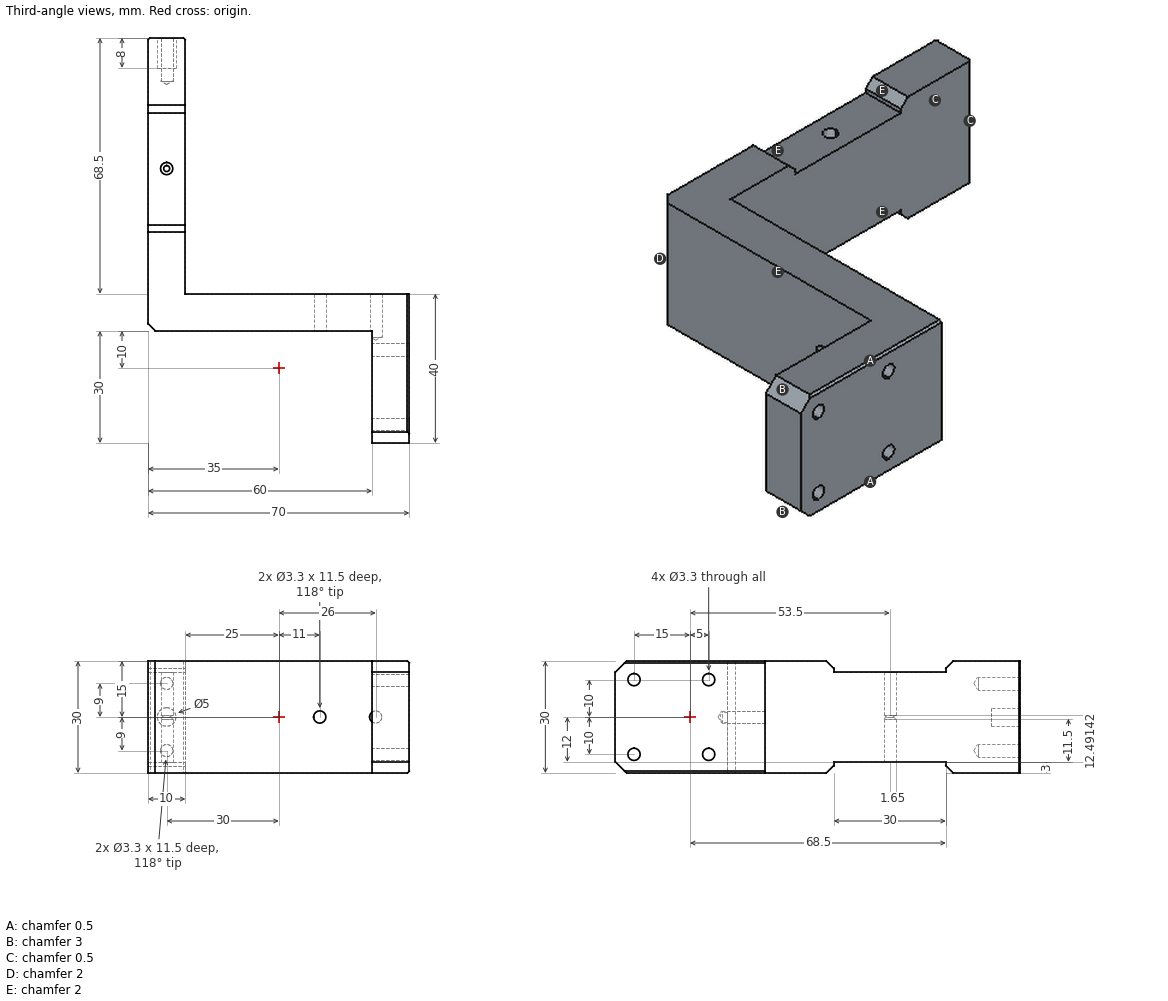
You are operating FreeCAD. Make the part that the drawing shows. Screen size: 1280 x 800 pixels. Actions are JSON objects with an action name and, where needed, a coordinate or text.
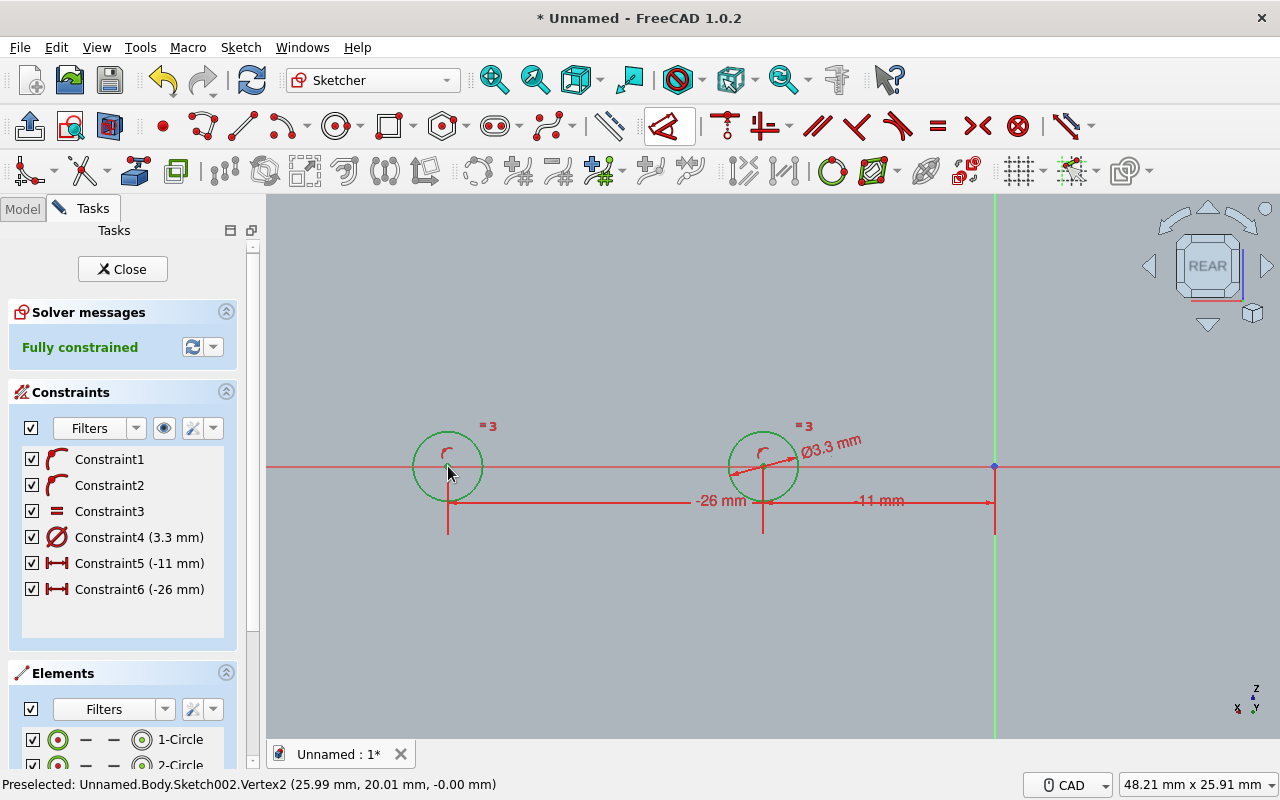
{"action": "left_click", "coordinate": [123, 269]}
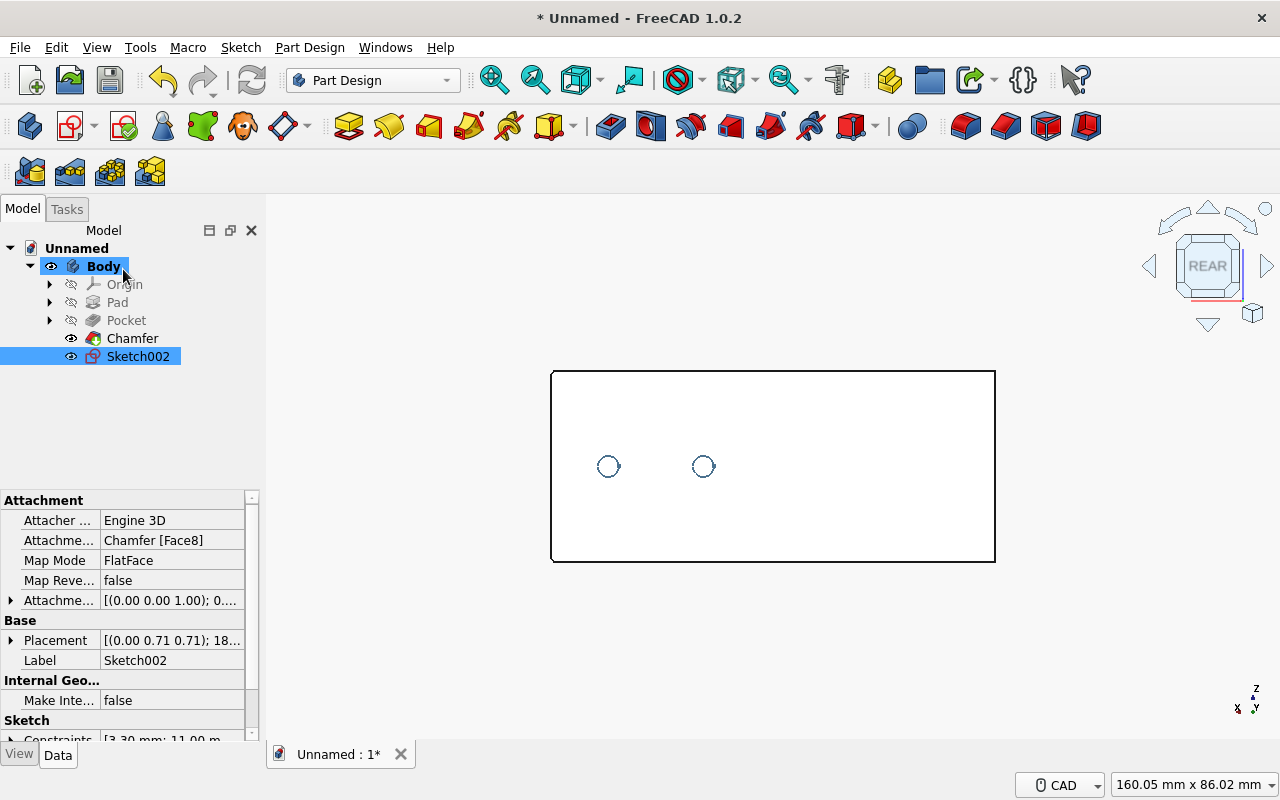
{"action": "left_click", "coordinate": [652, 126]}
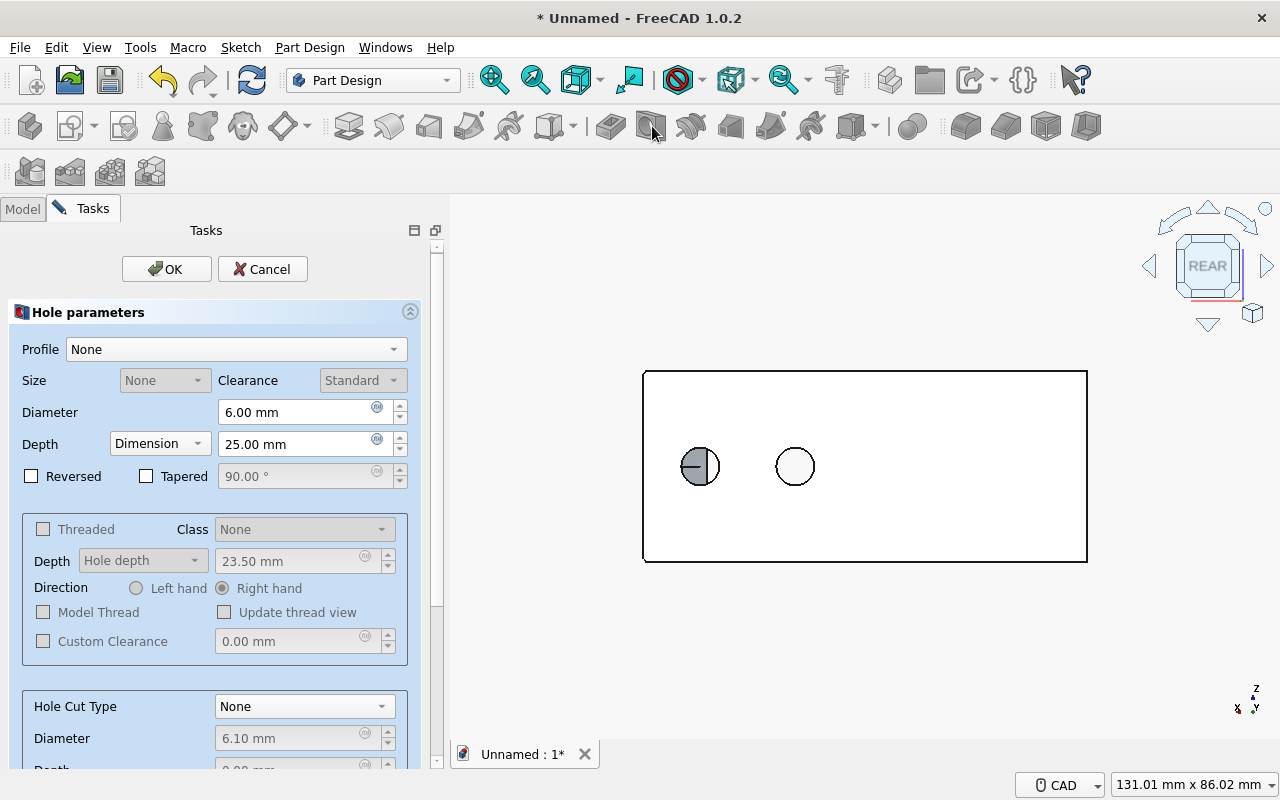
{"action": "triple_click", "coordinate": [305, 412]}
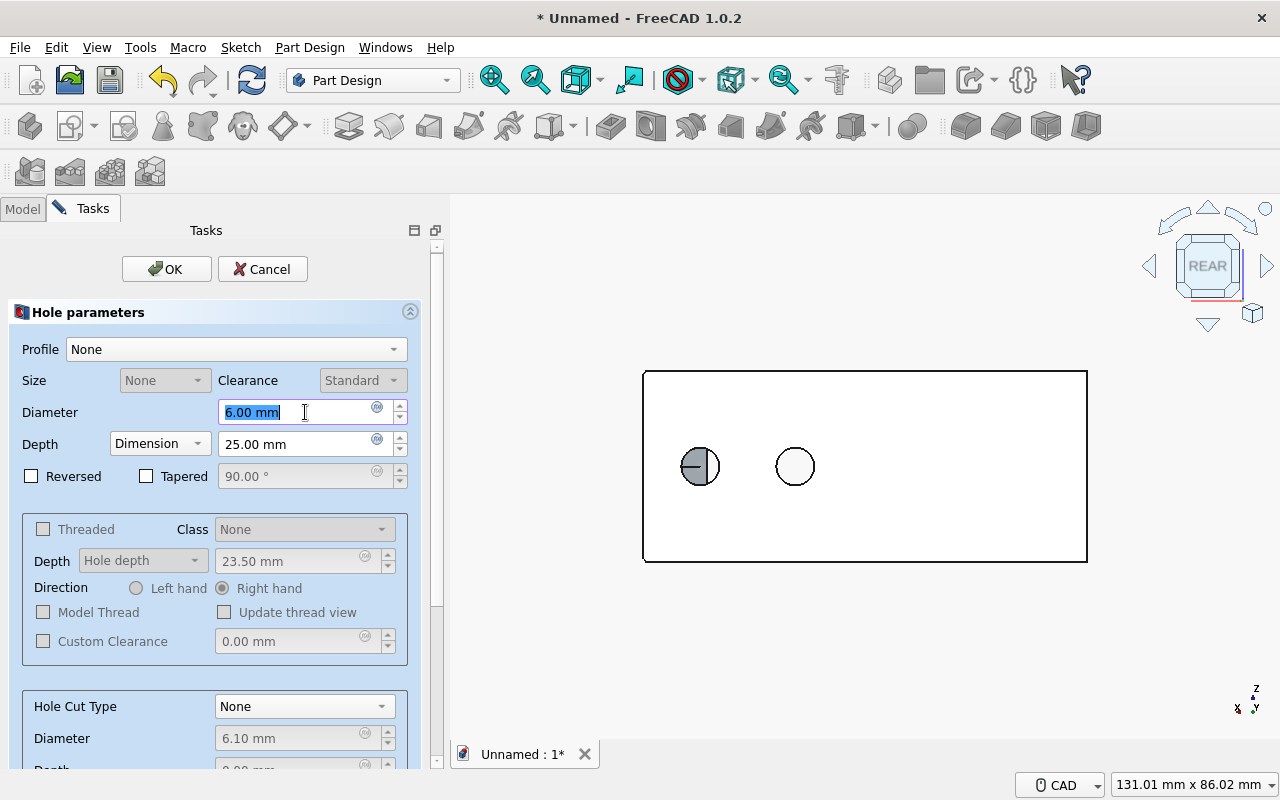
{"action": "type", "text": "3.3"}
{"action": "key", "text": "Tab"}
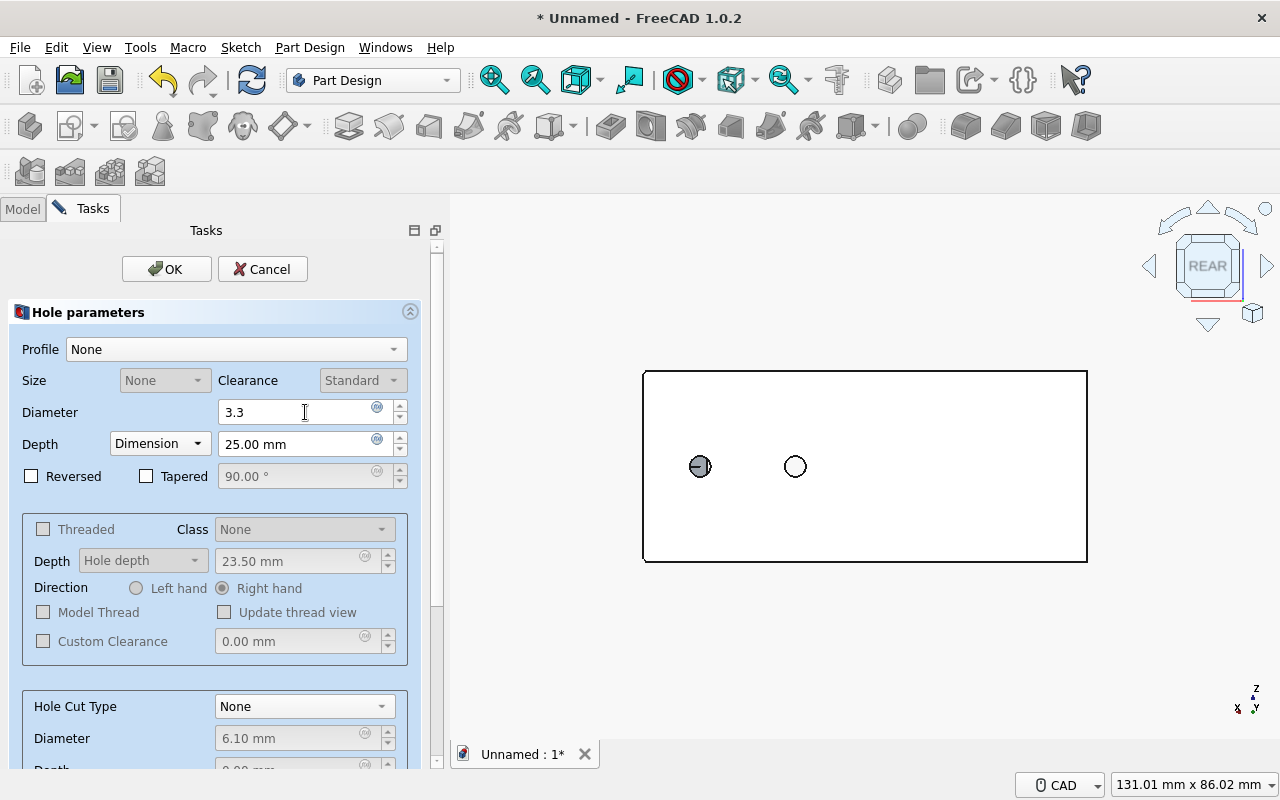
{"action": "triple_click", "coordinate": [305, 444]}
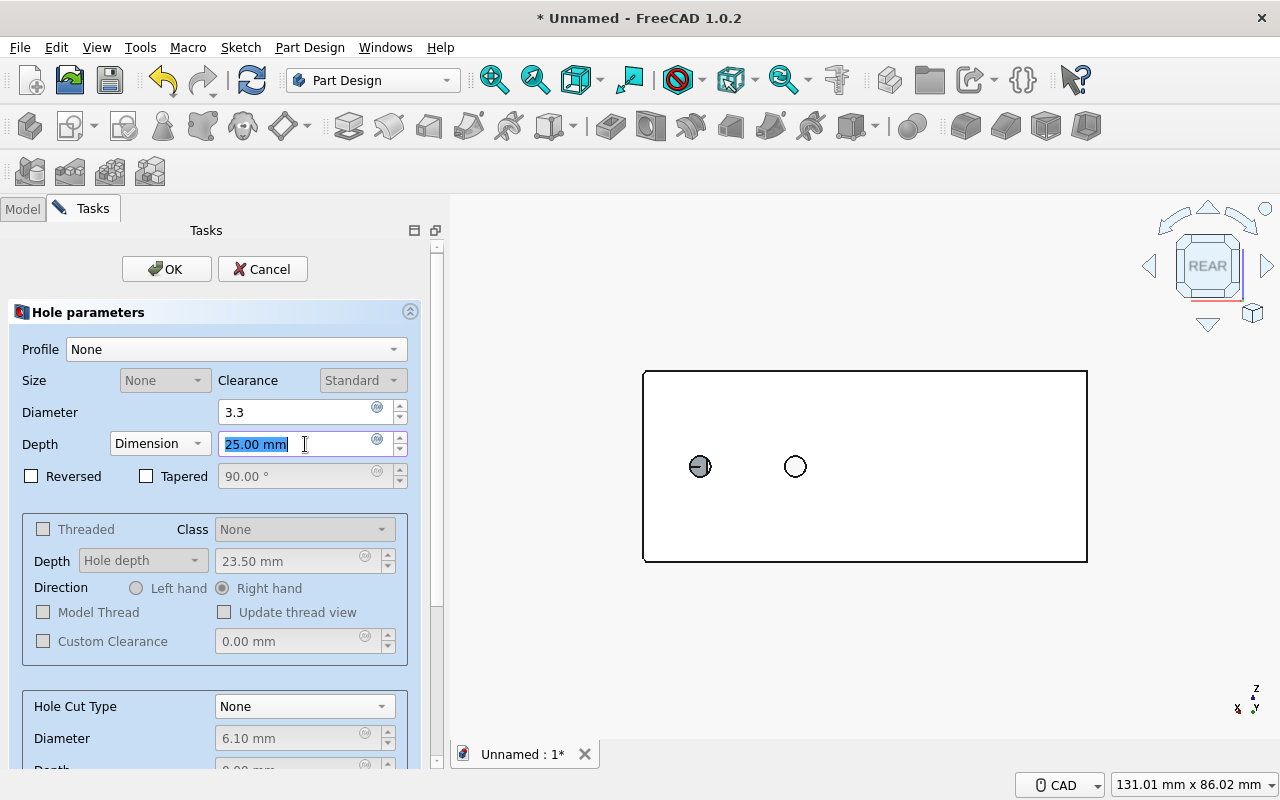
{"action": "type", "text": "11.5"}
{"action": "key", "text": "Tab"}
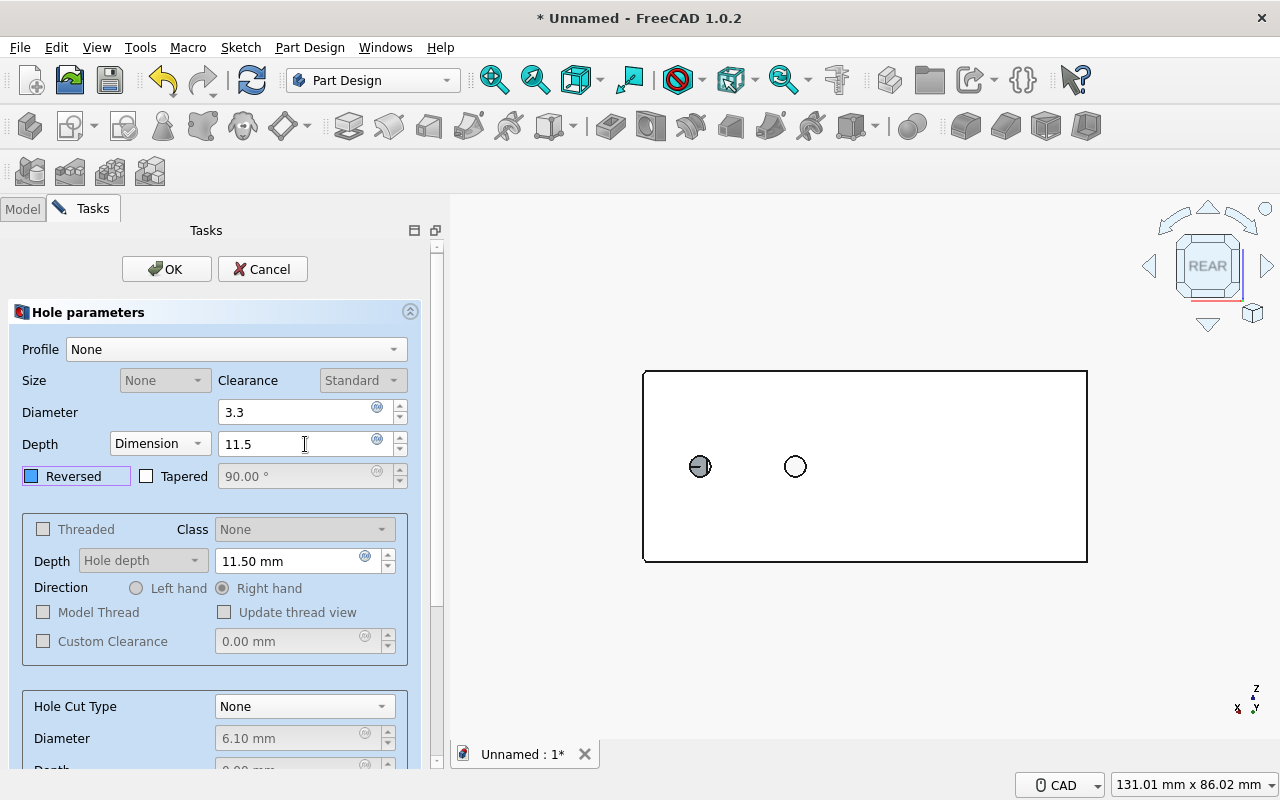
{"action": "left_click", "coordinate": [167, 269]}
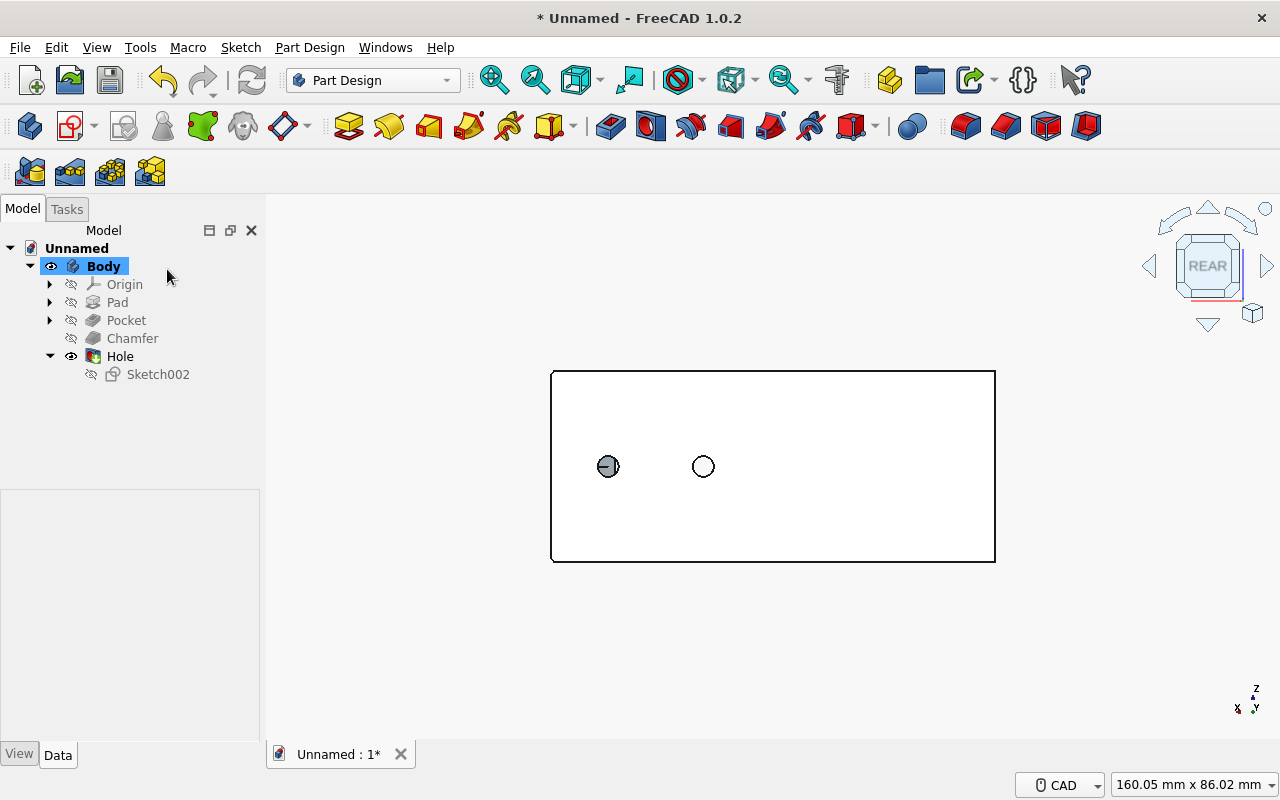
{"action": "left_click", "coordinate": [496, 80]}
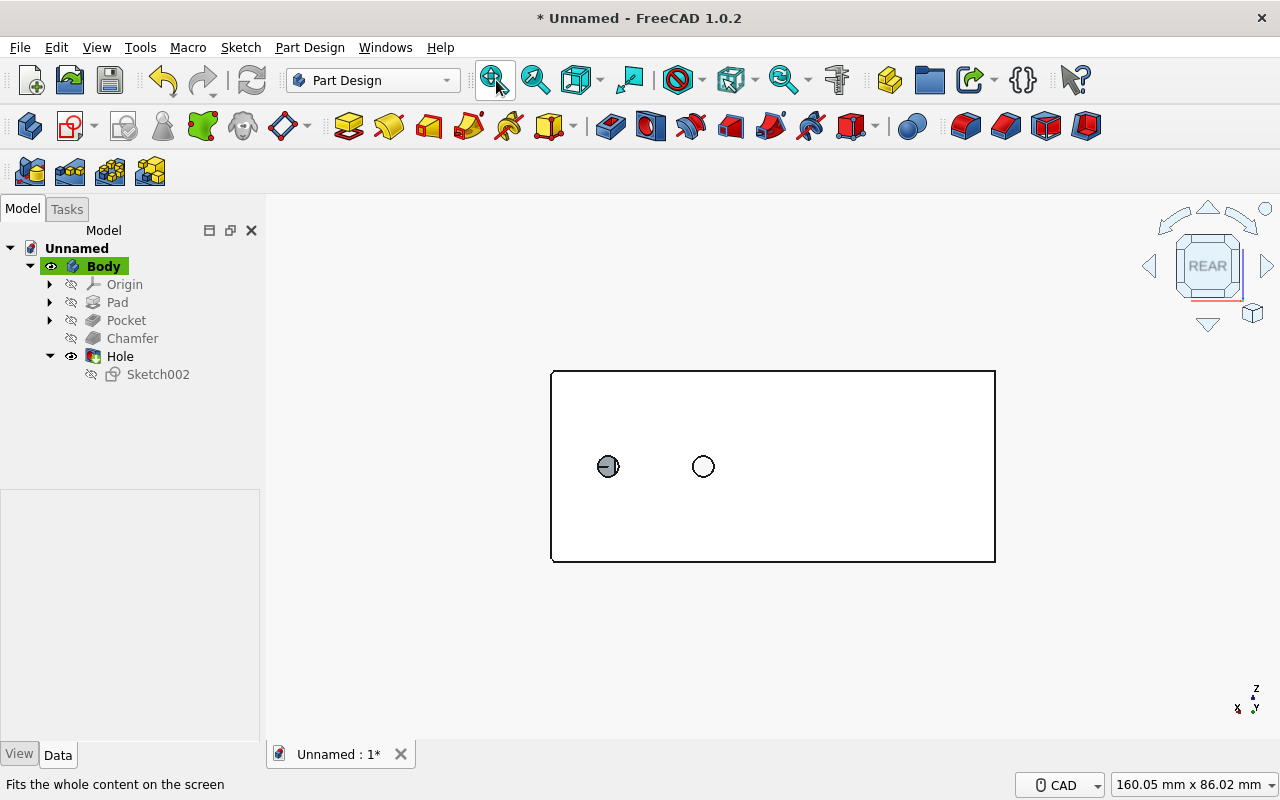
{"action": "key", "text": "0"}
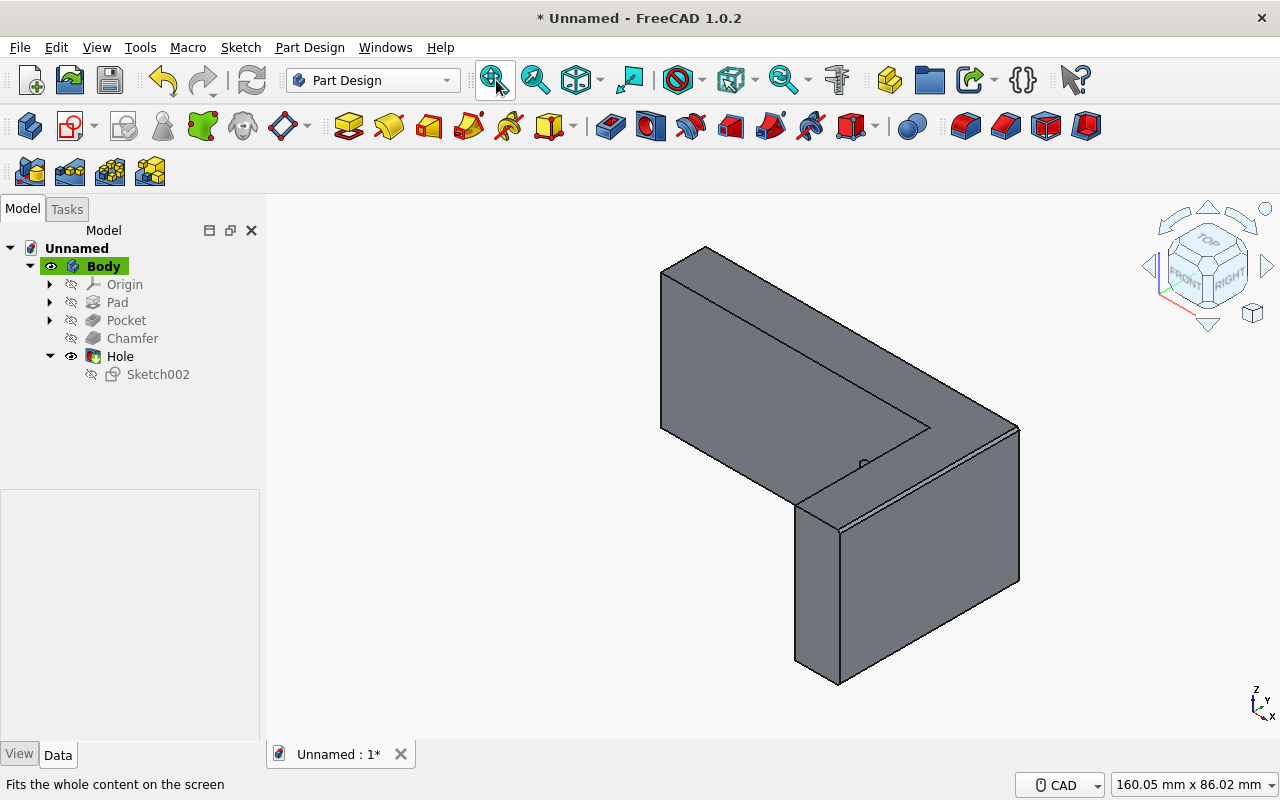
{"action": "left_click", "coordinate": [930, 556]}